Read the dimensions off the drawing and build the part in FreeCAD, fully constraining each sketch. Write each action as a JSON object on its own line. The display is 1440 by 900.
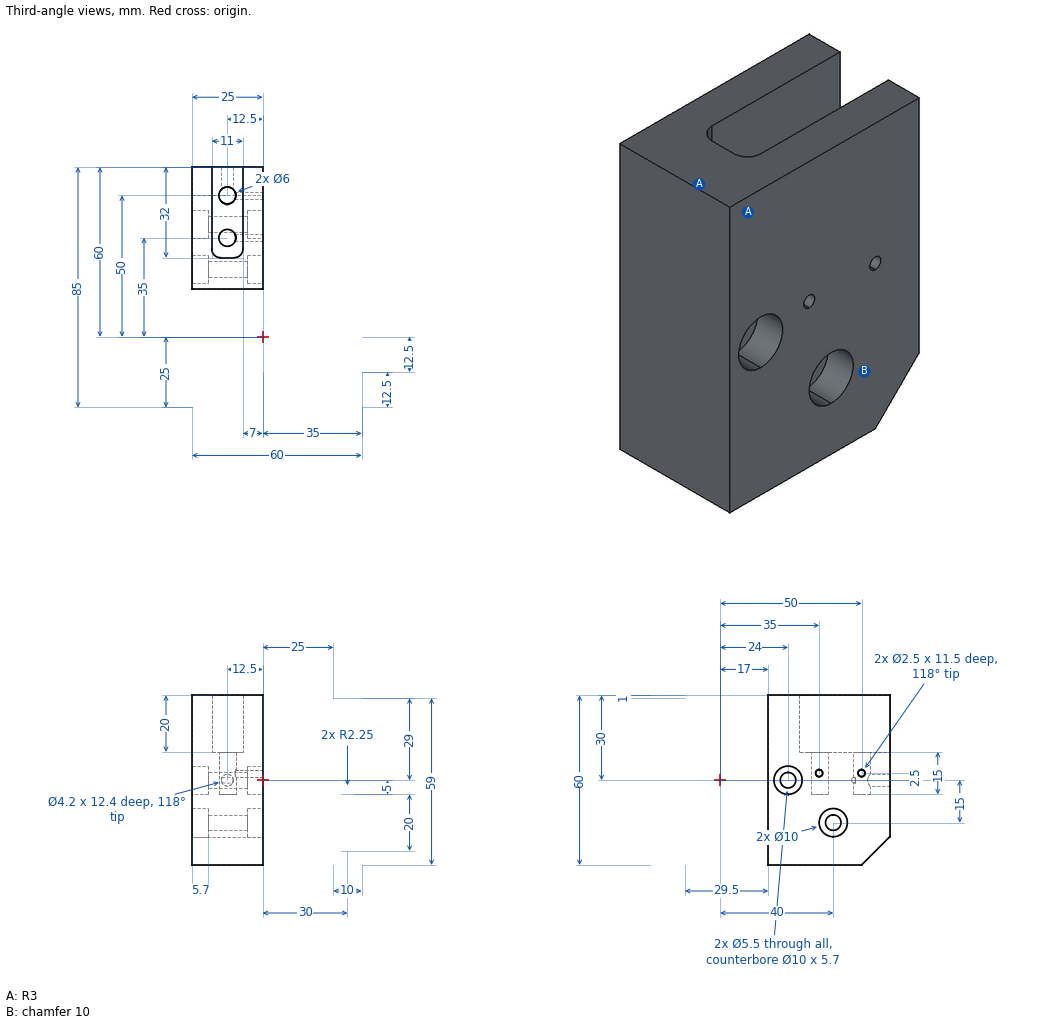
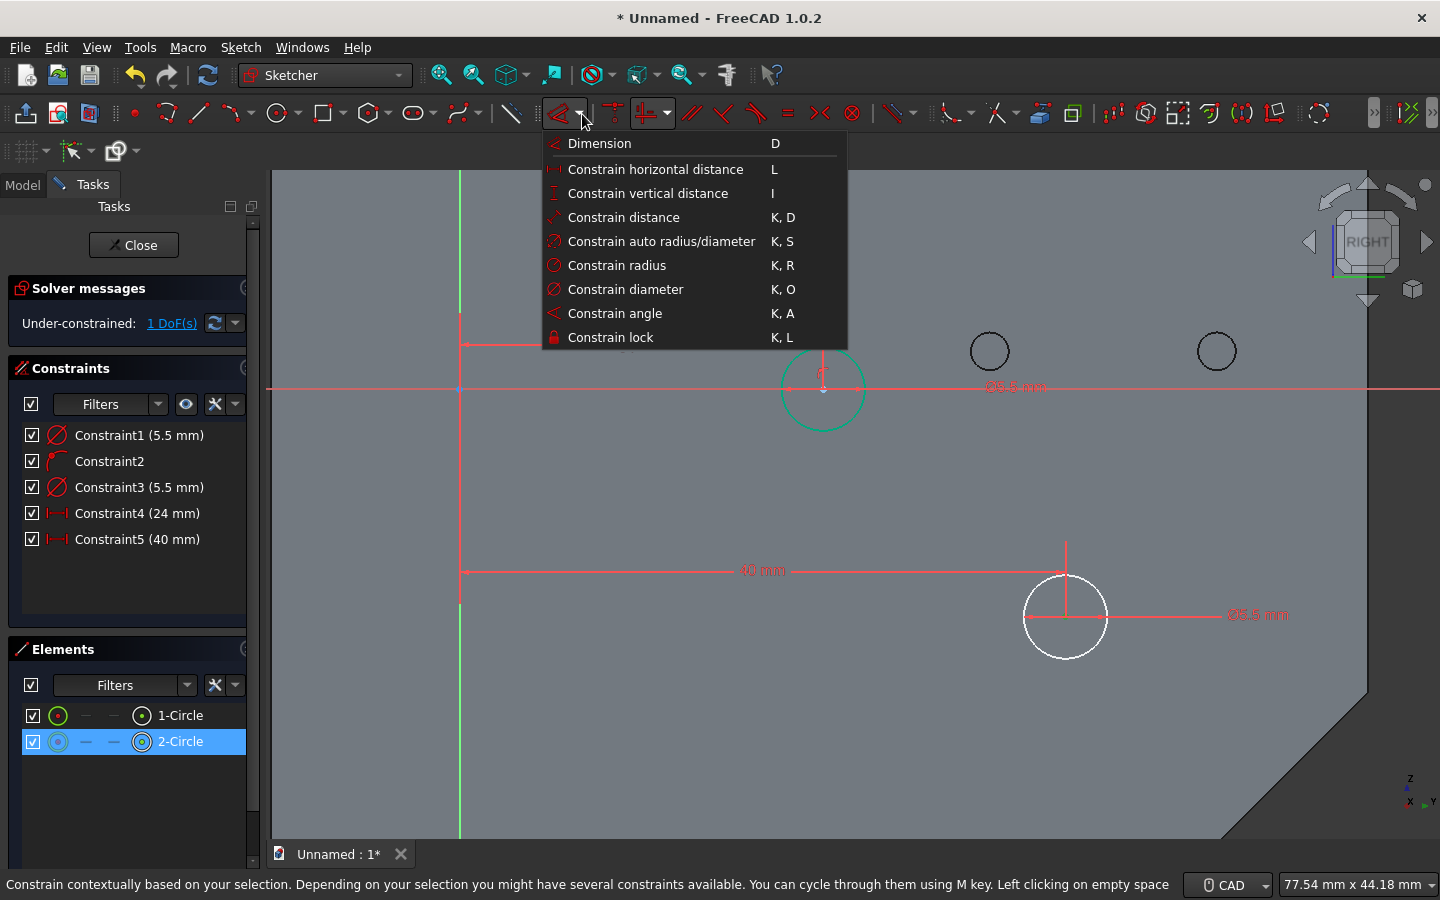
{"action": "left_click", "coordinate": [695, 193]}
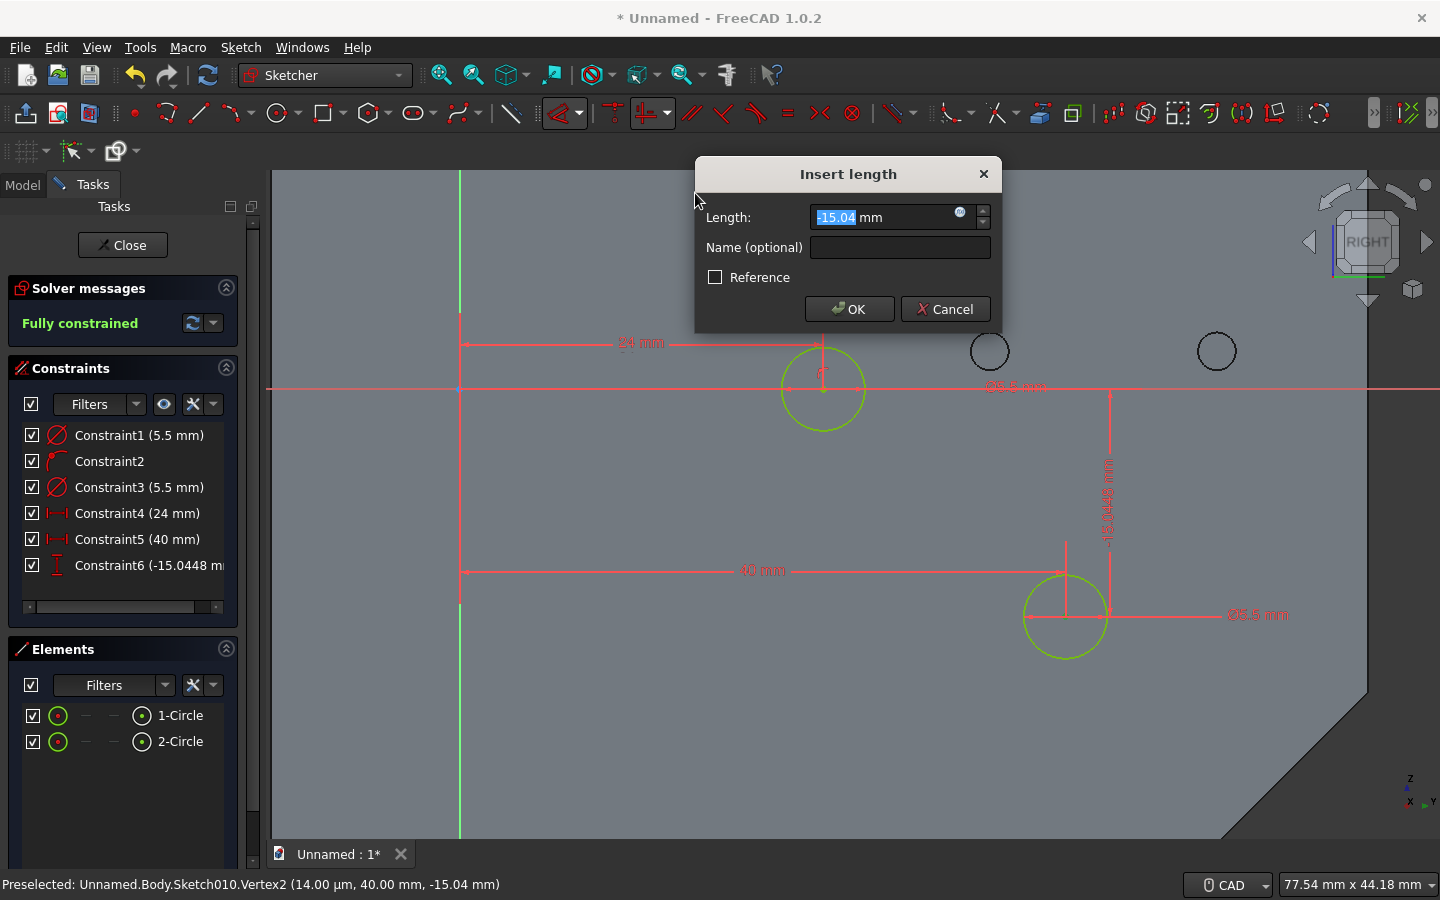
{"action": "type", "text": "-15"}
{"action": "key", "text": "Return"}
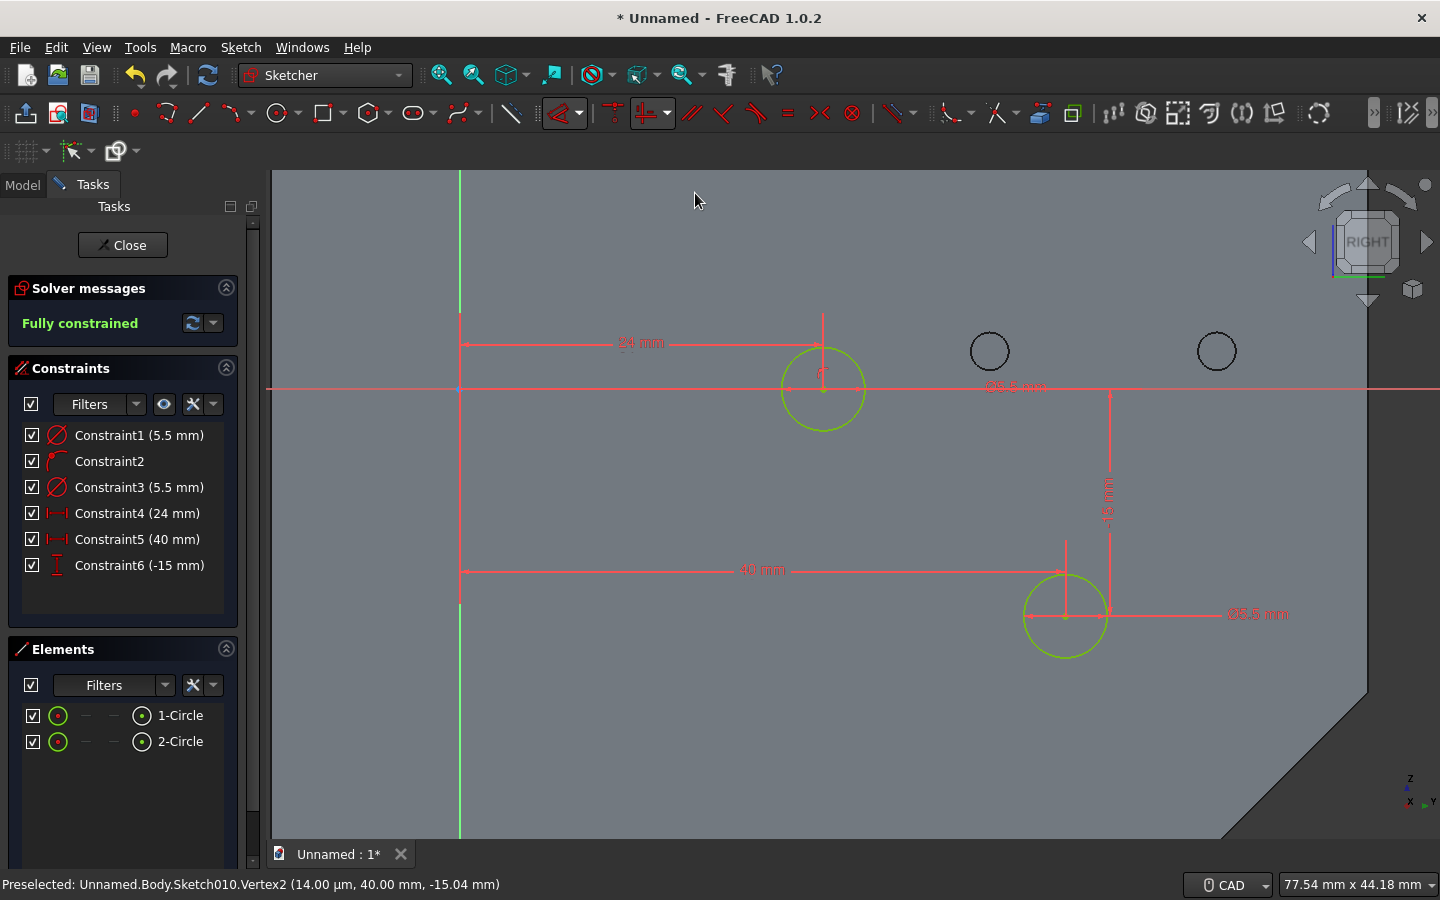
{"action": "left_click", "coordinate": [123, 245]}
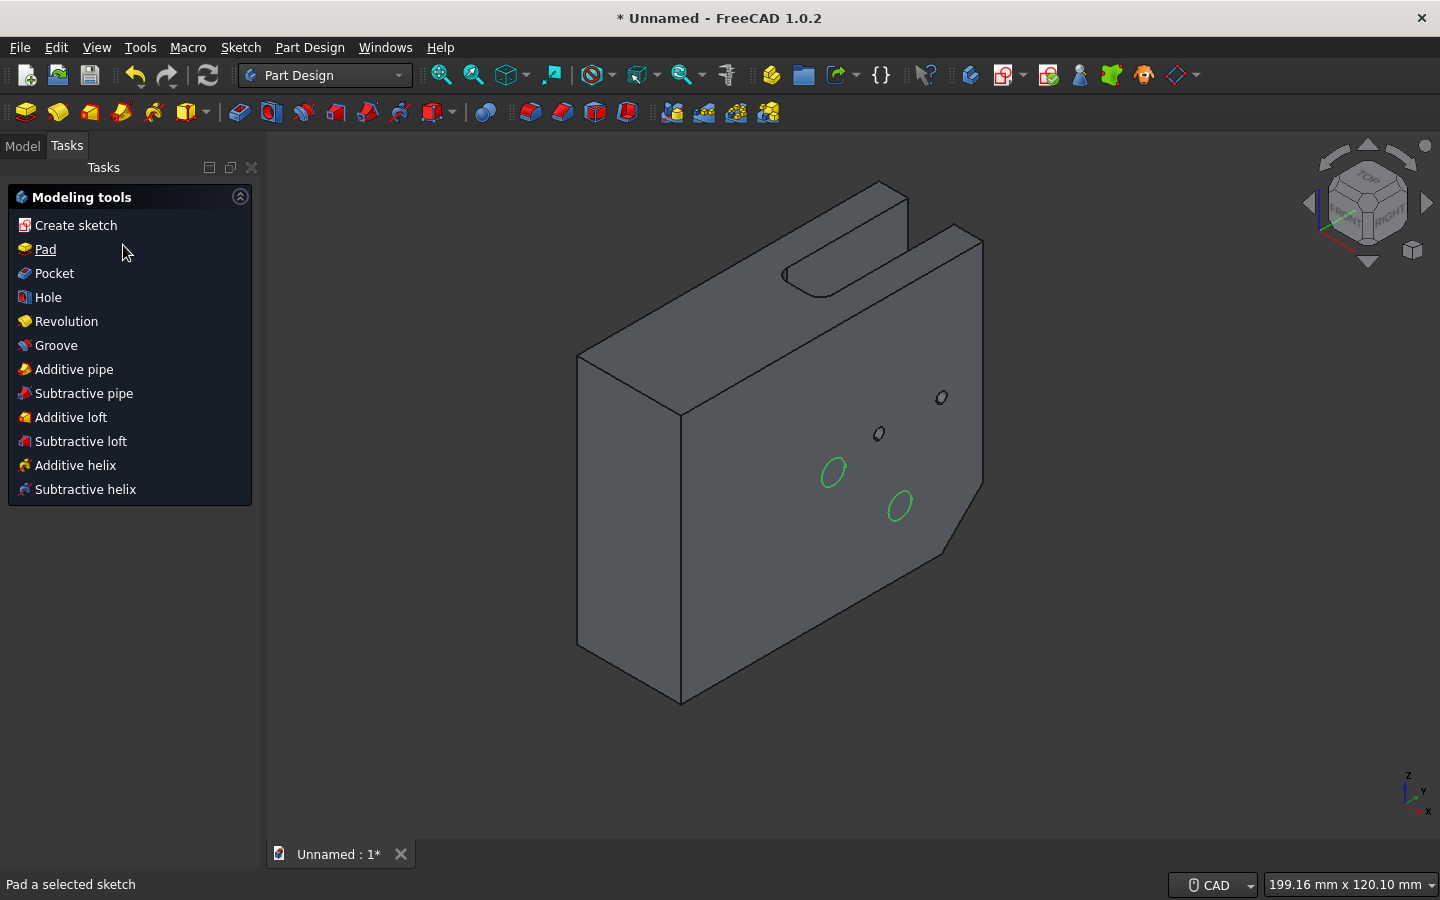
{"action": "left_click", "coordinate": [272, 112]}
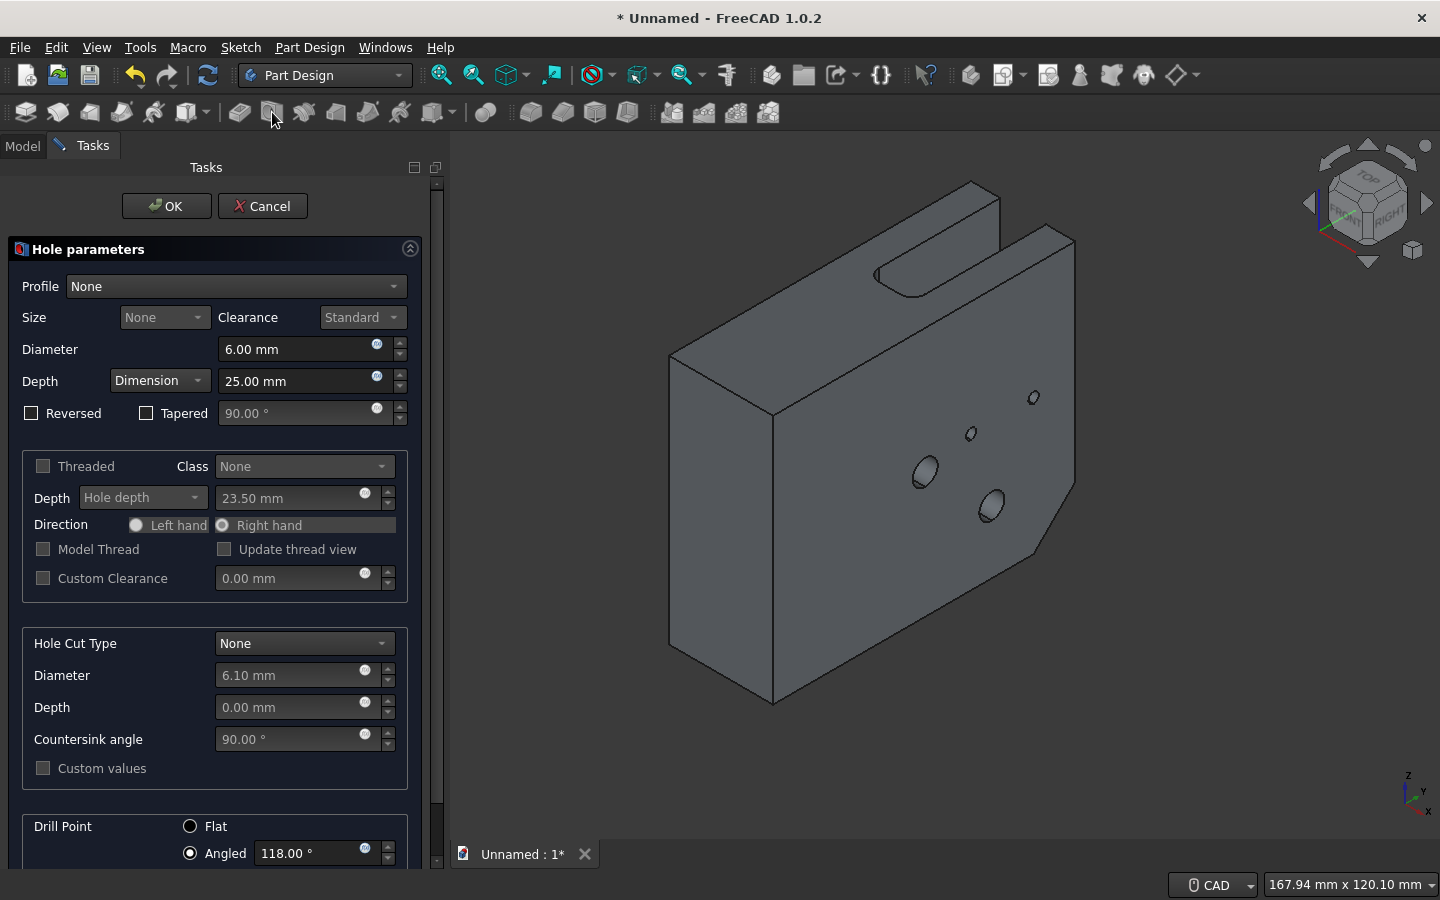
{"action": "triple_click", "coordinate": [305, 349]}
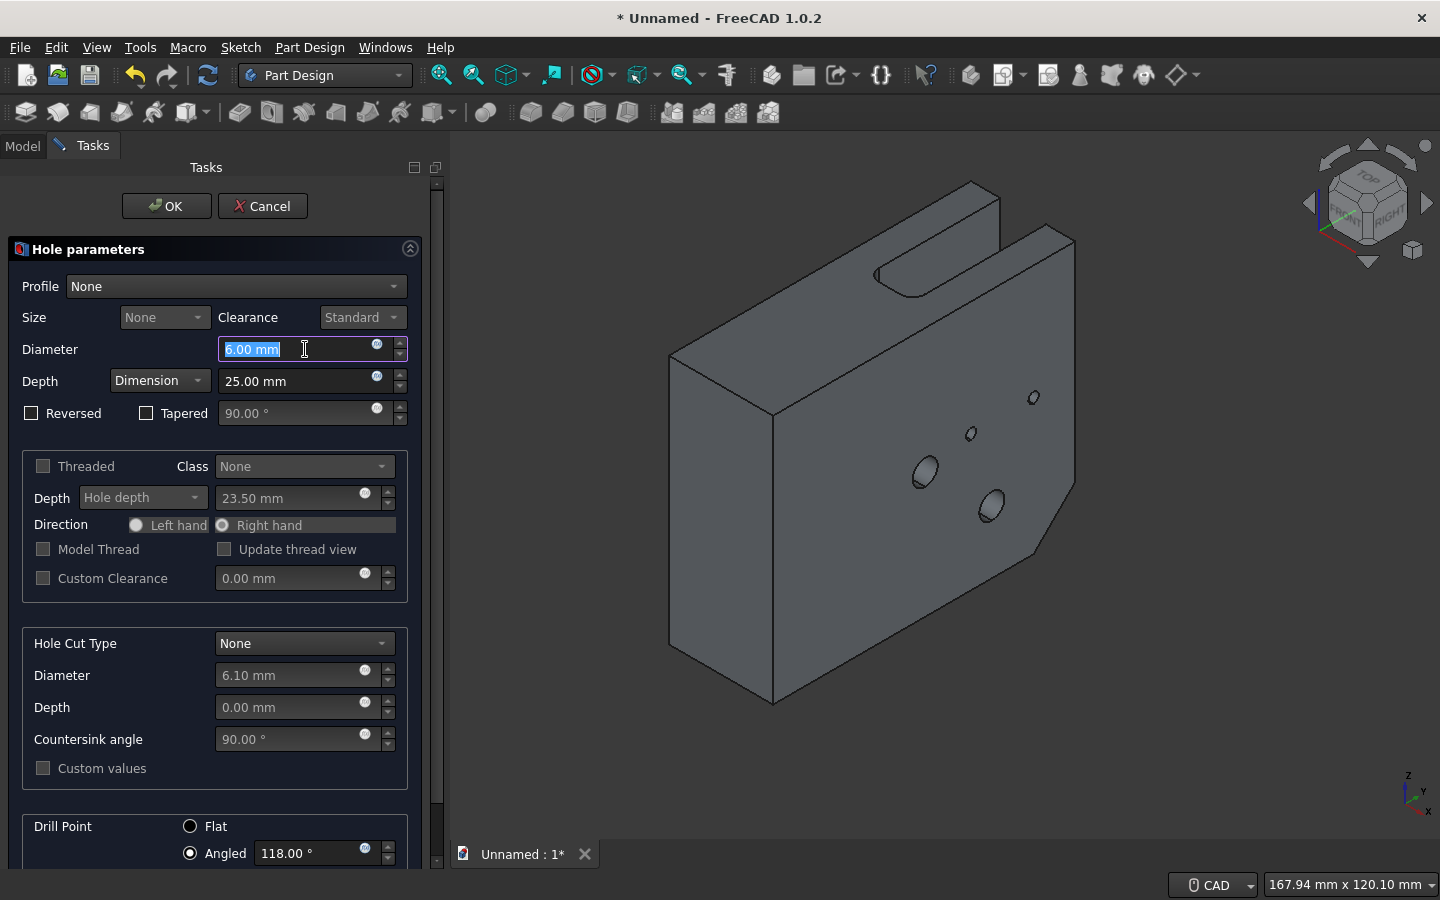
{"action": "type", "text": "5.5"}
{"action": "key", "text": "Tab"}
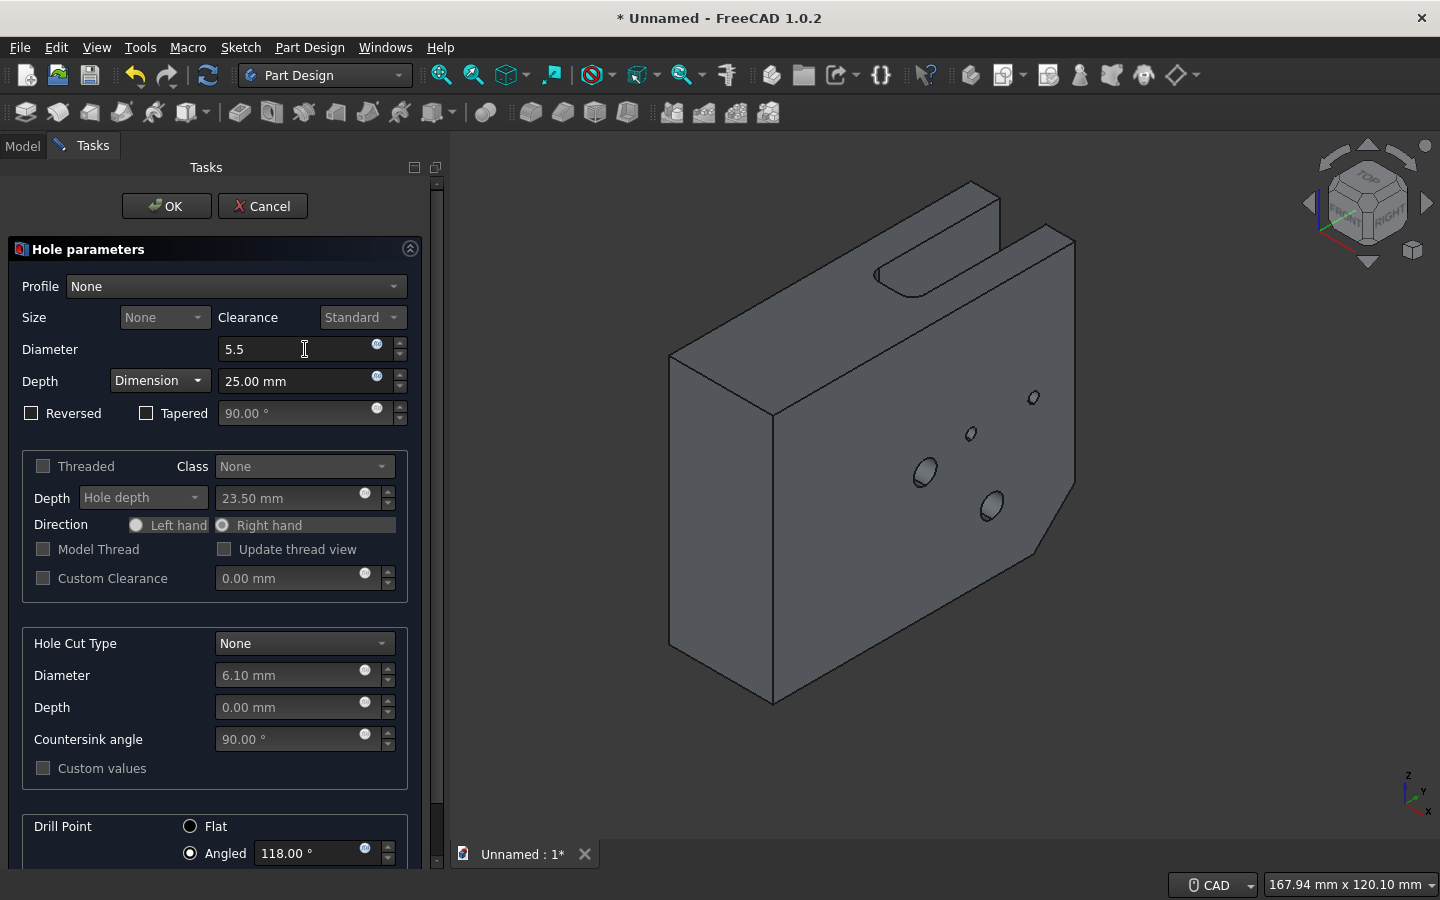
{"action": "left_click", "coordinate": [161, 380]}